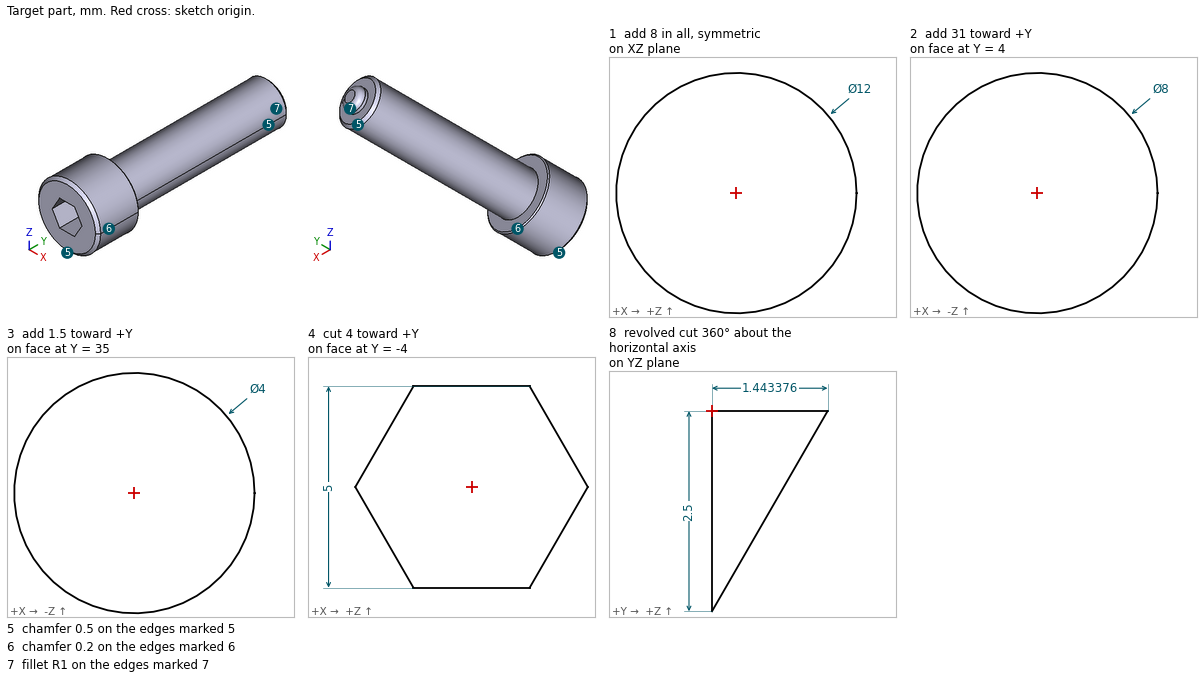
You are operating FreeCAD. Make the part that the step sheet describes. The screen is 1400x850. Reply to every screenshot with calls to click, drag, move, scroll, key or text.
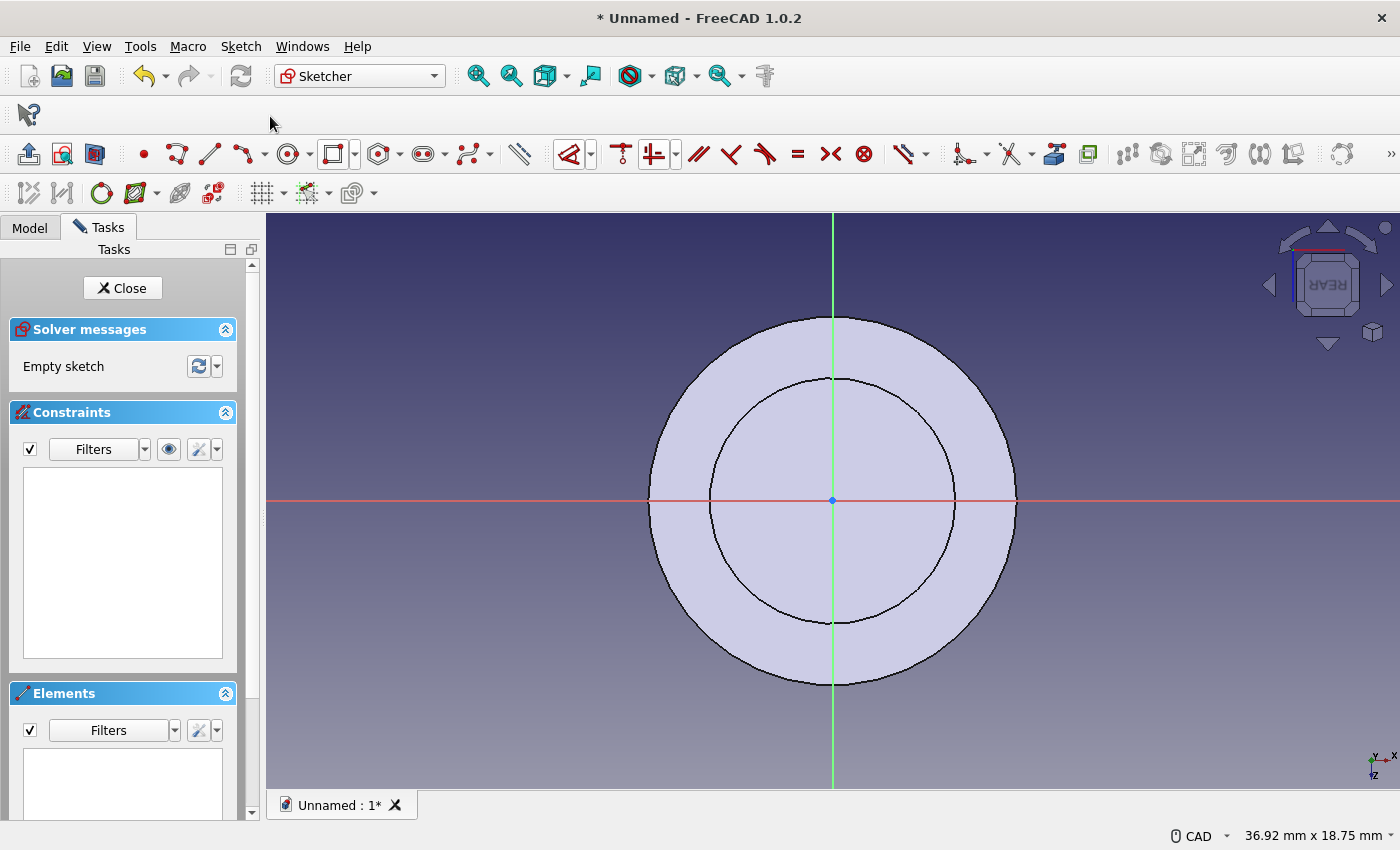
scroll(872, 501, up, 5)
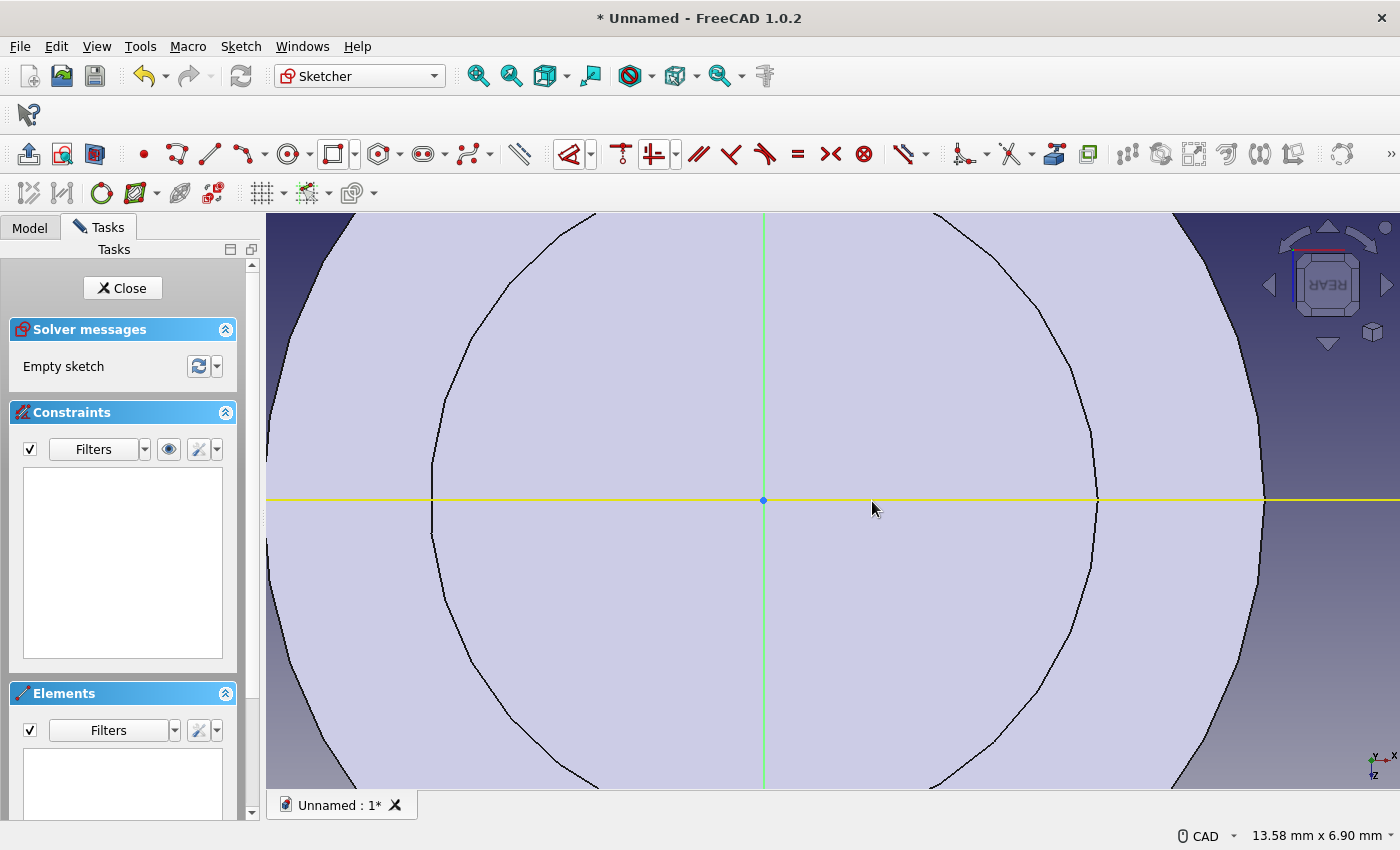
click(288, 154)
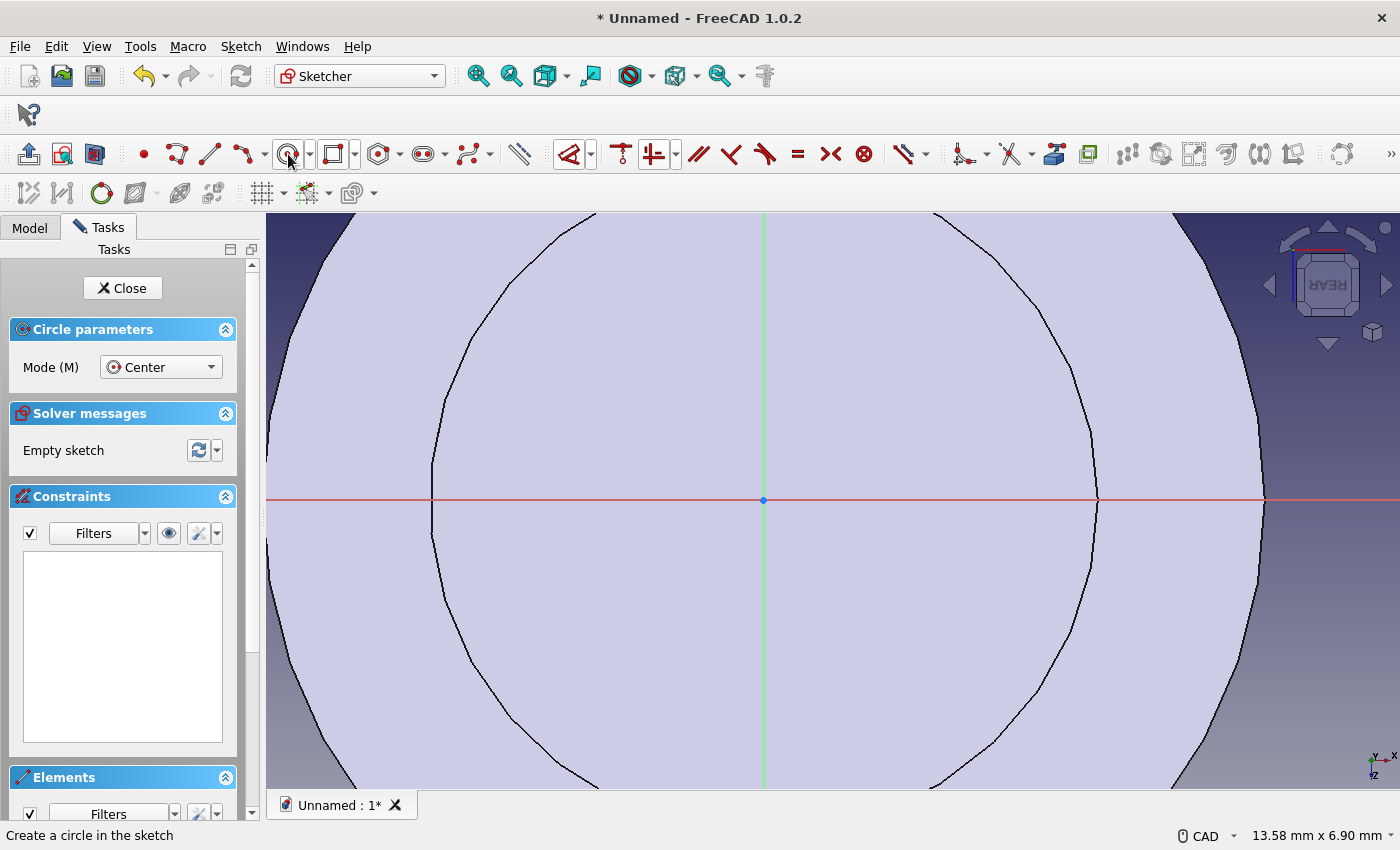
click(764, 500)
move(882, 382)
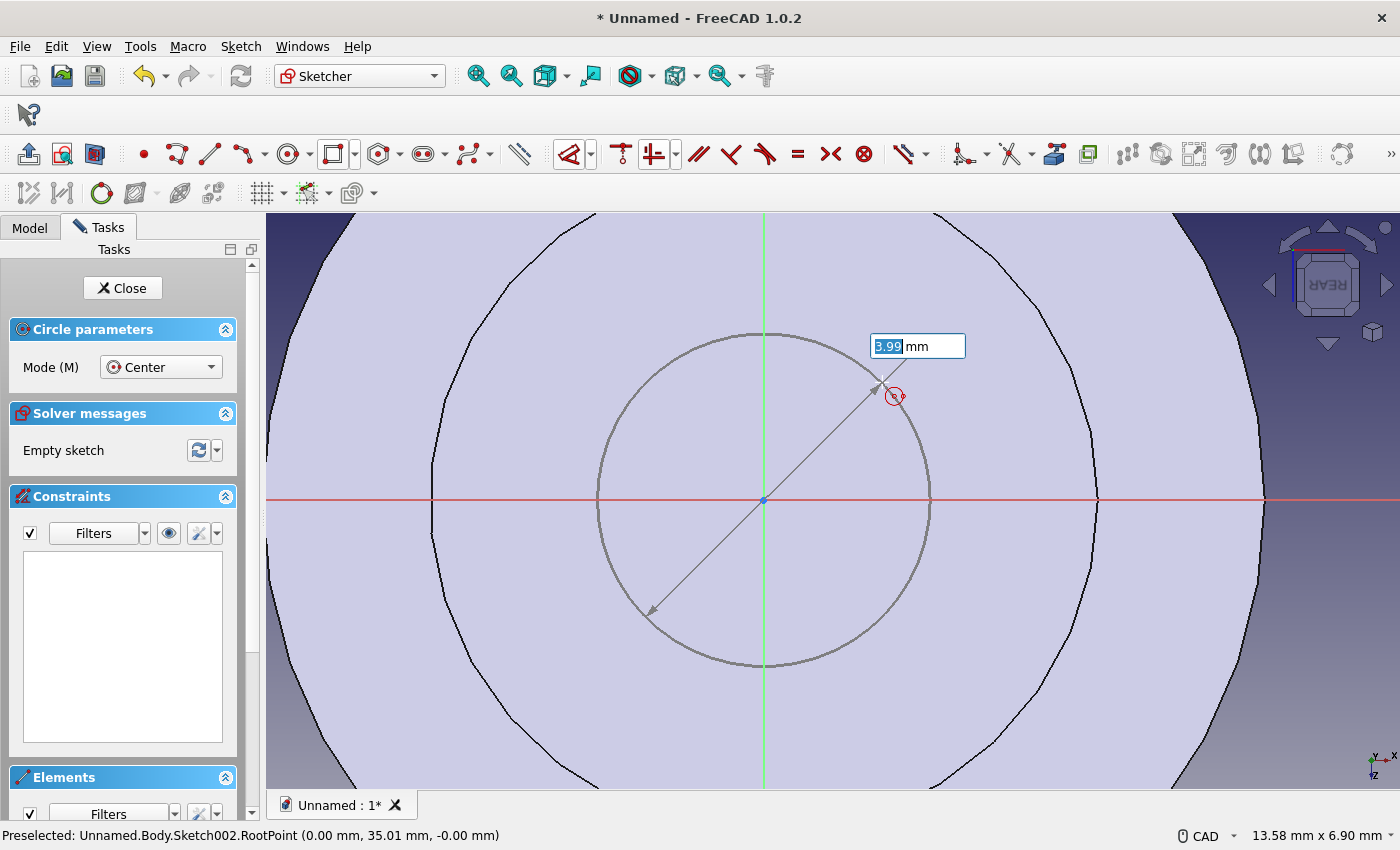
text(4)
key(Return)
key(Escape)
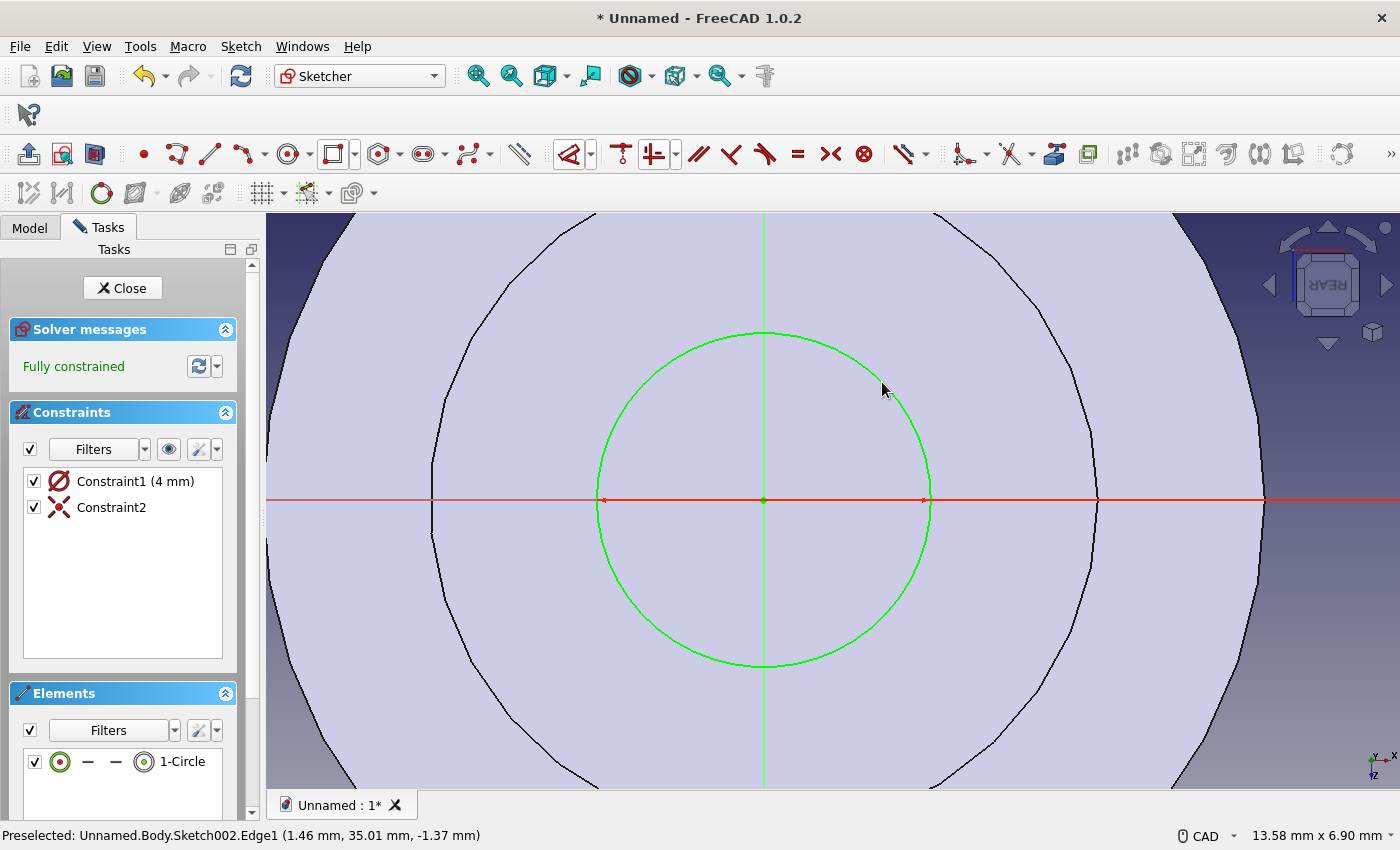
click(123, 288)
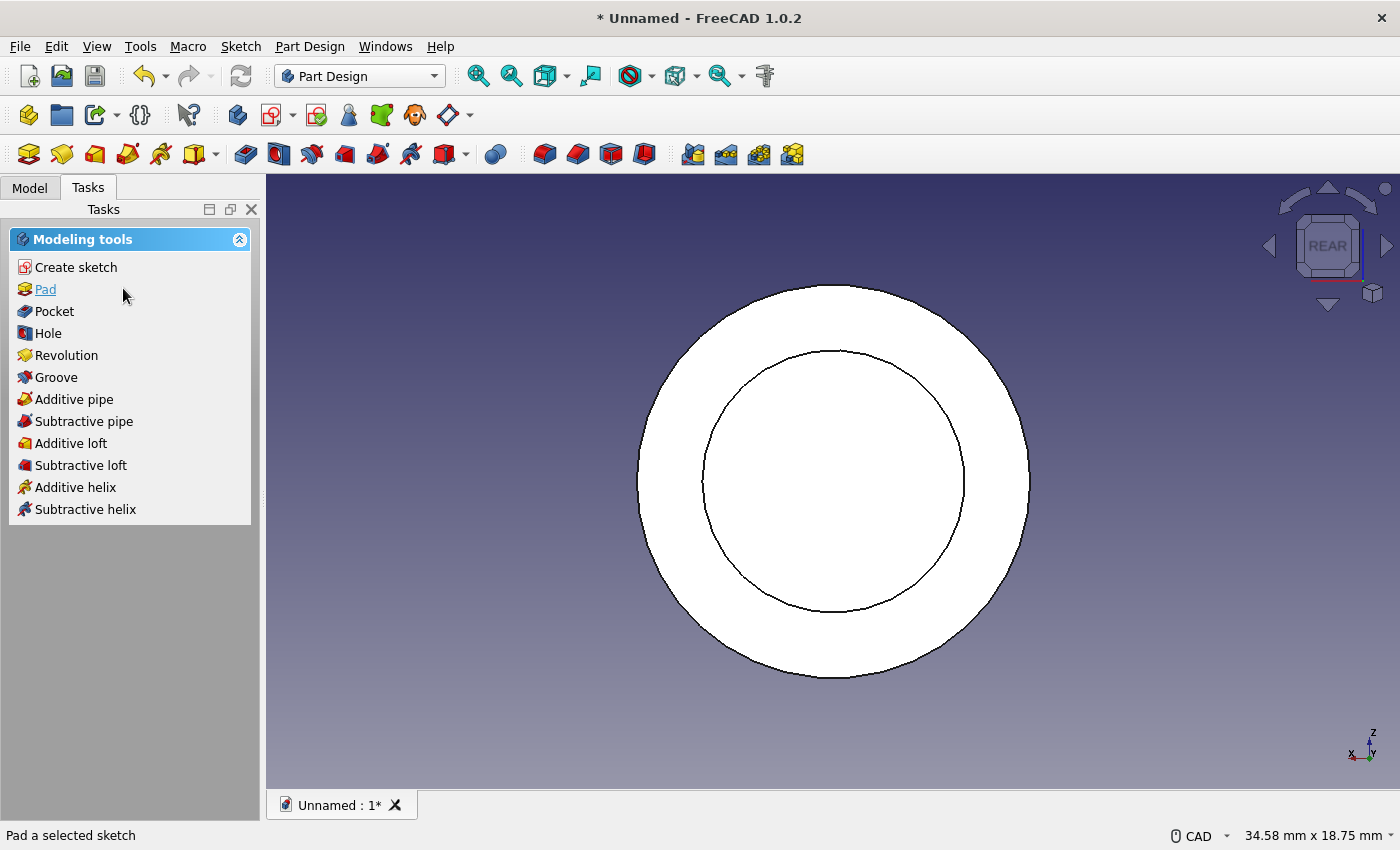
click(29, 154)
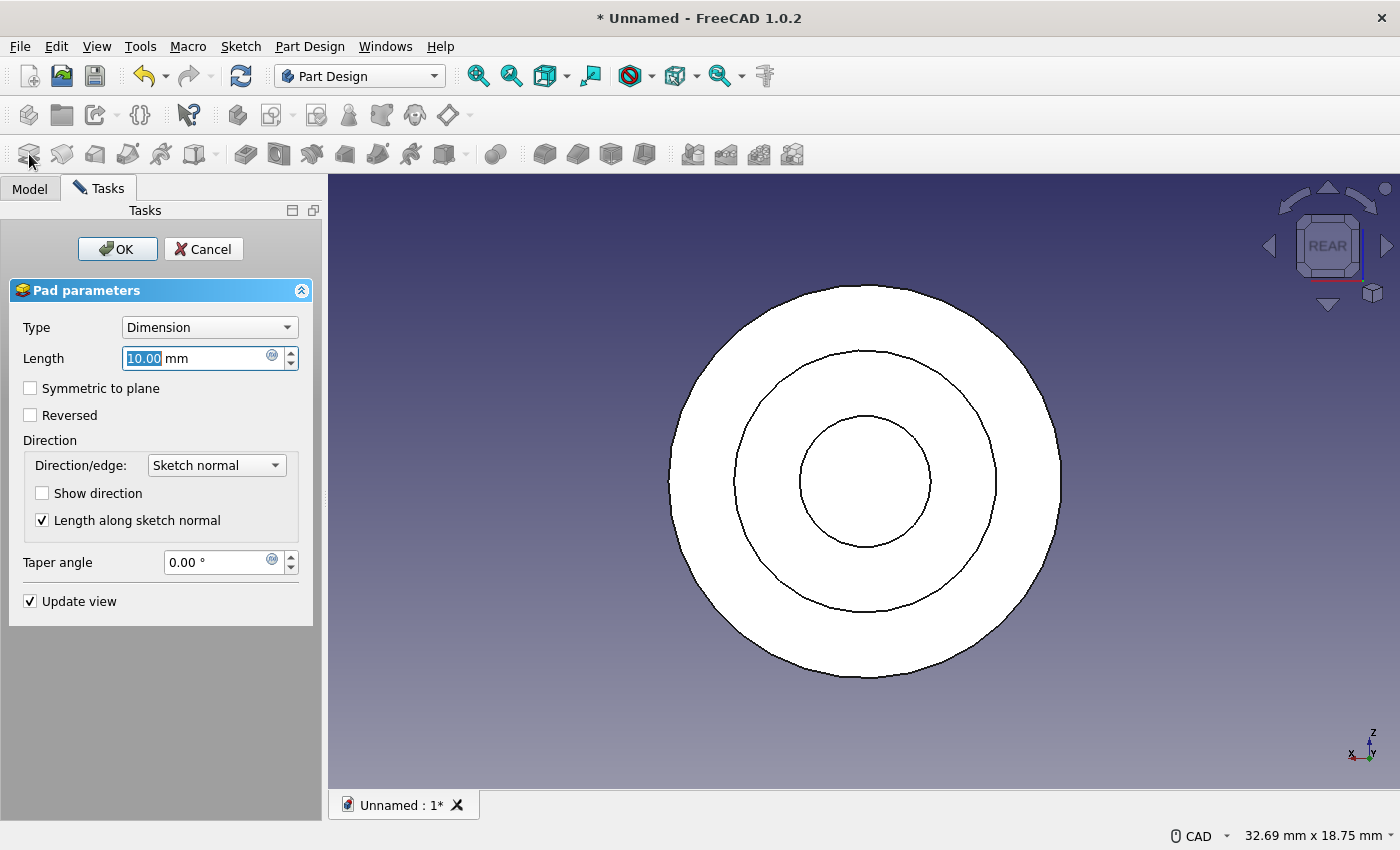
text(1.5)
key(Tab)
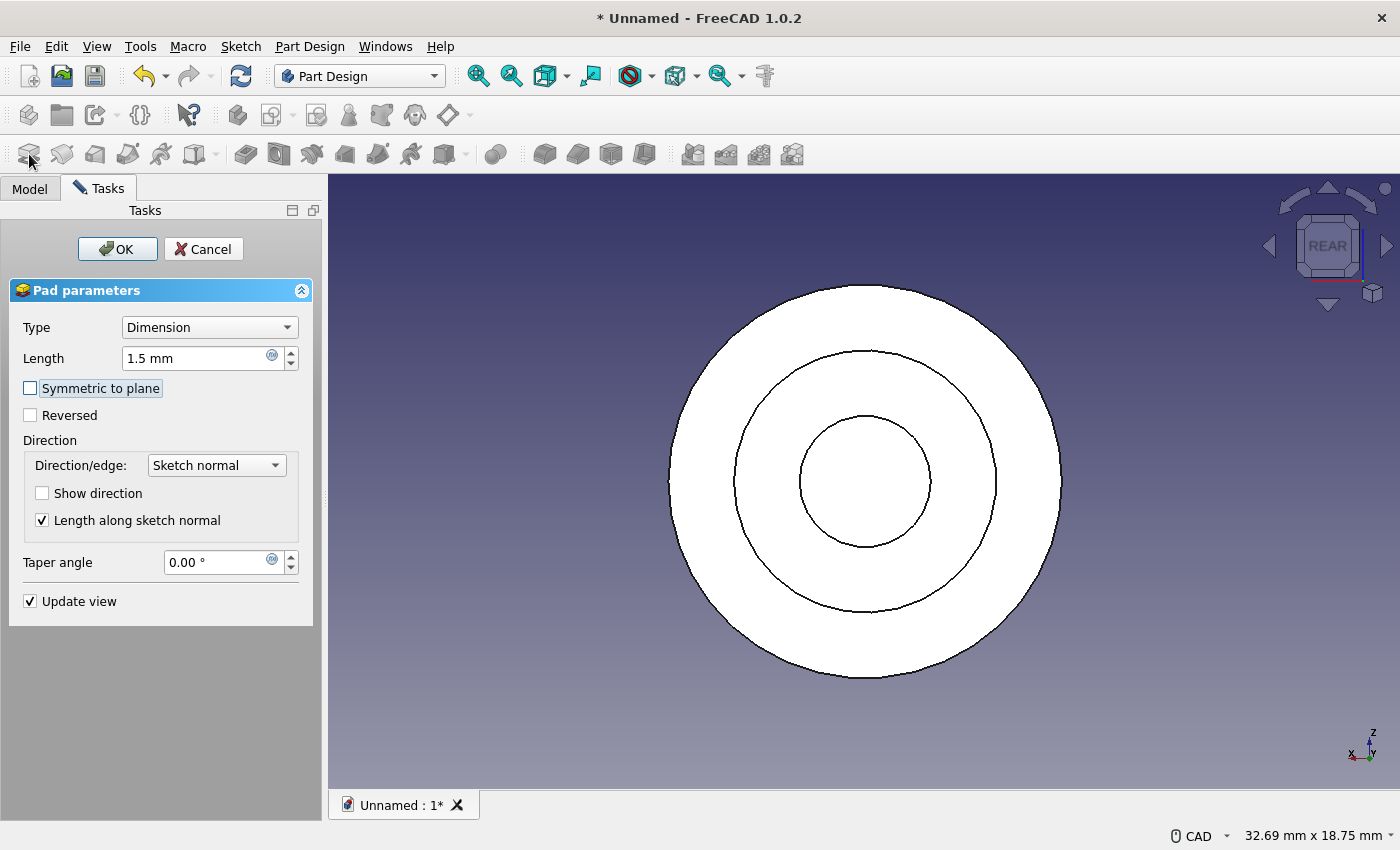
click(118, 249)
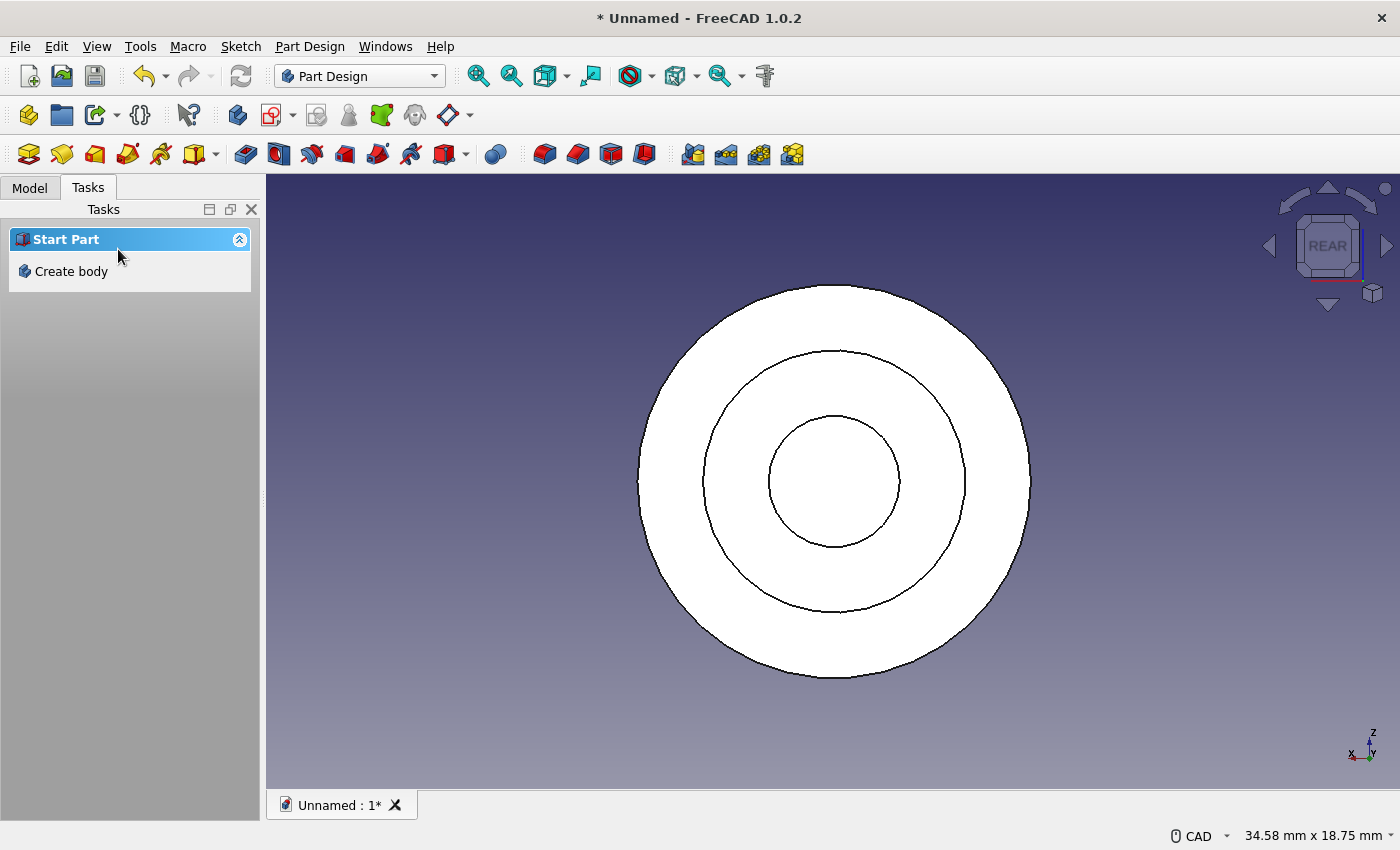
key(0)